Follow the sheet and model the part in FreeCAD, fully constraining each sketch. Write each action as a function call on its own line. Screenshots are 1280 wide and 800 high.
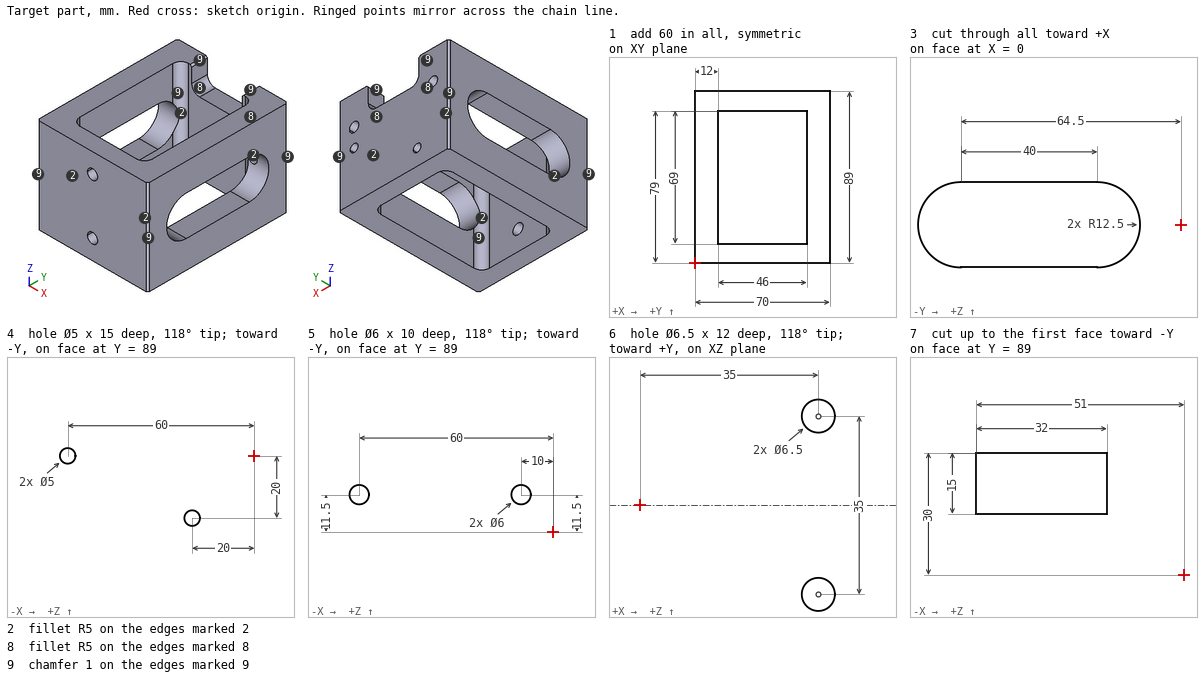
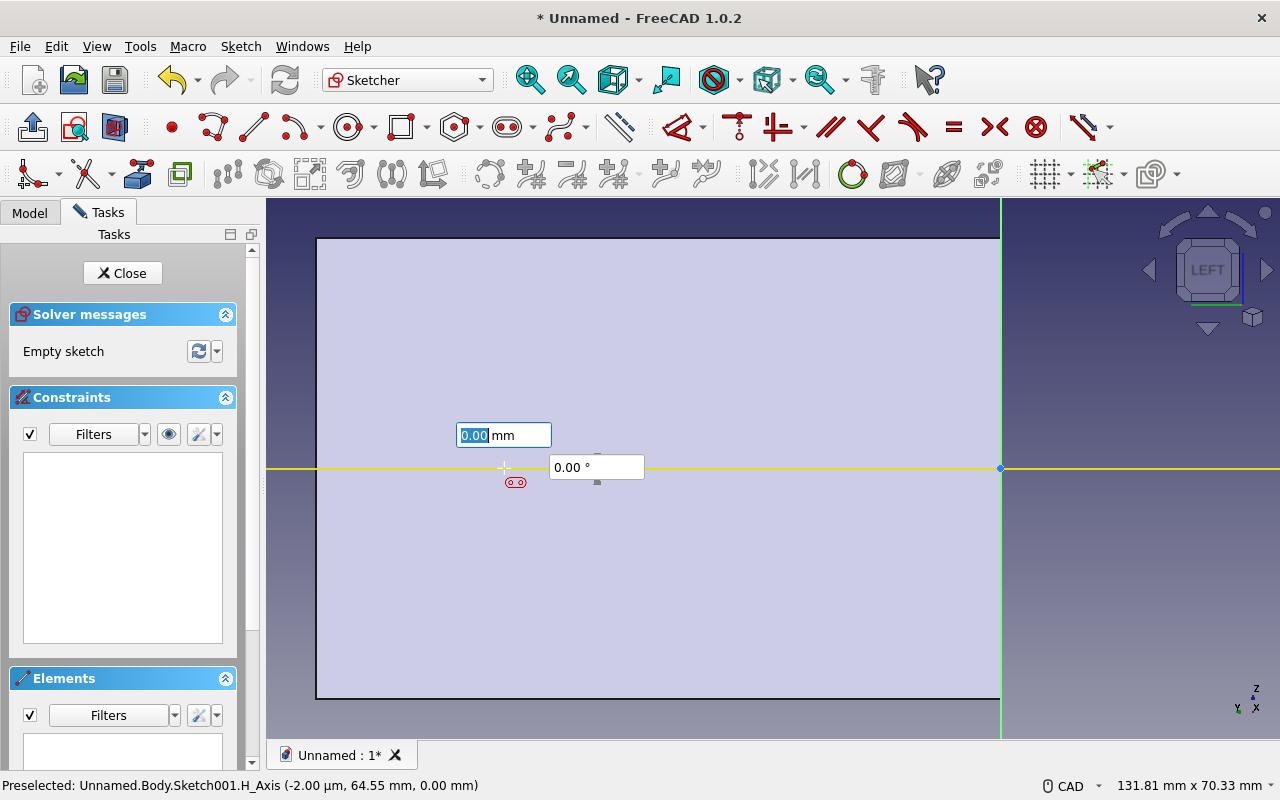
click(812, 459)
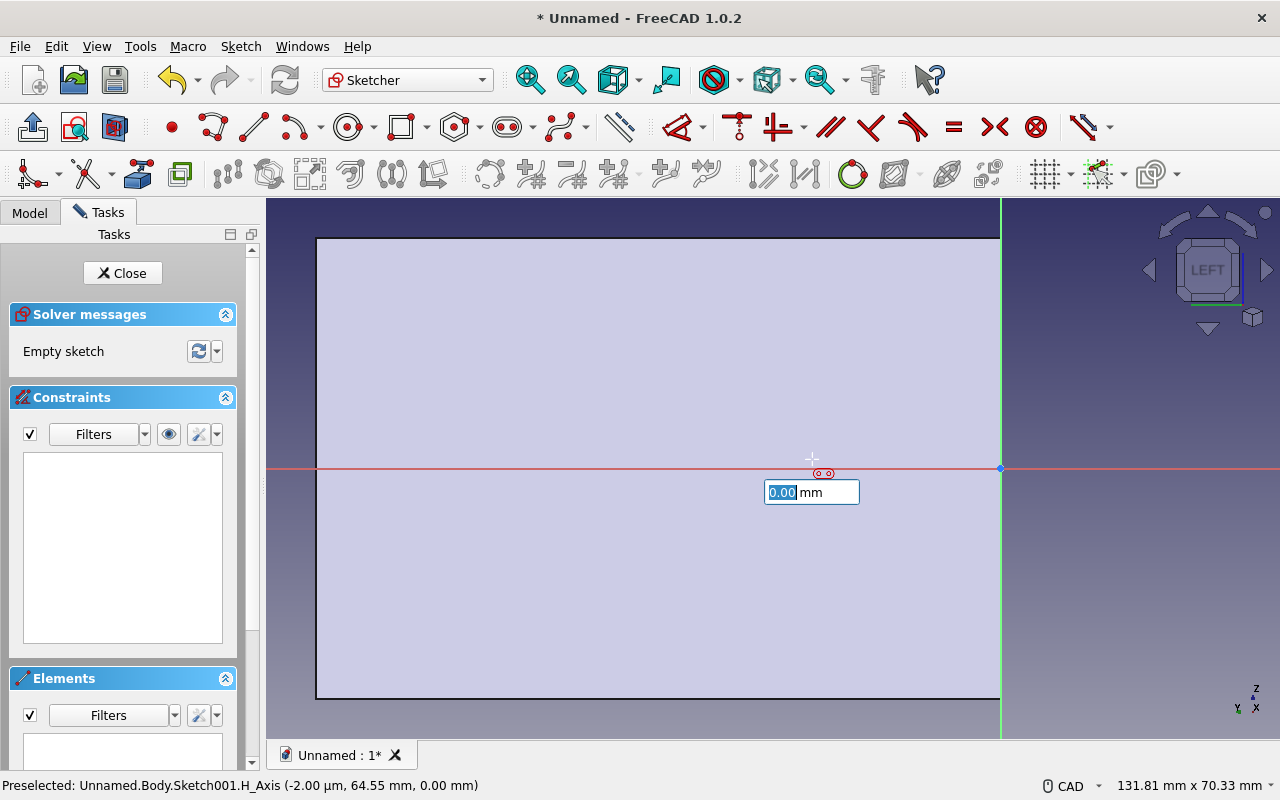
click(658, 565)
key(Escape)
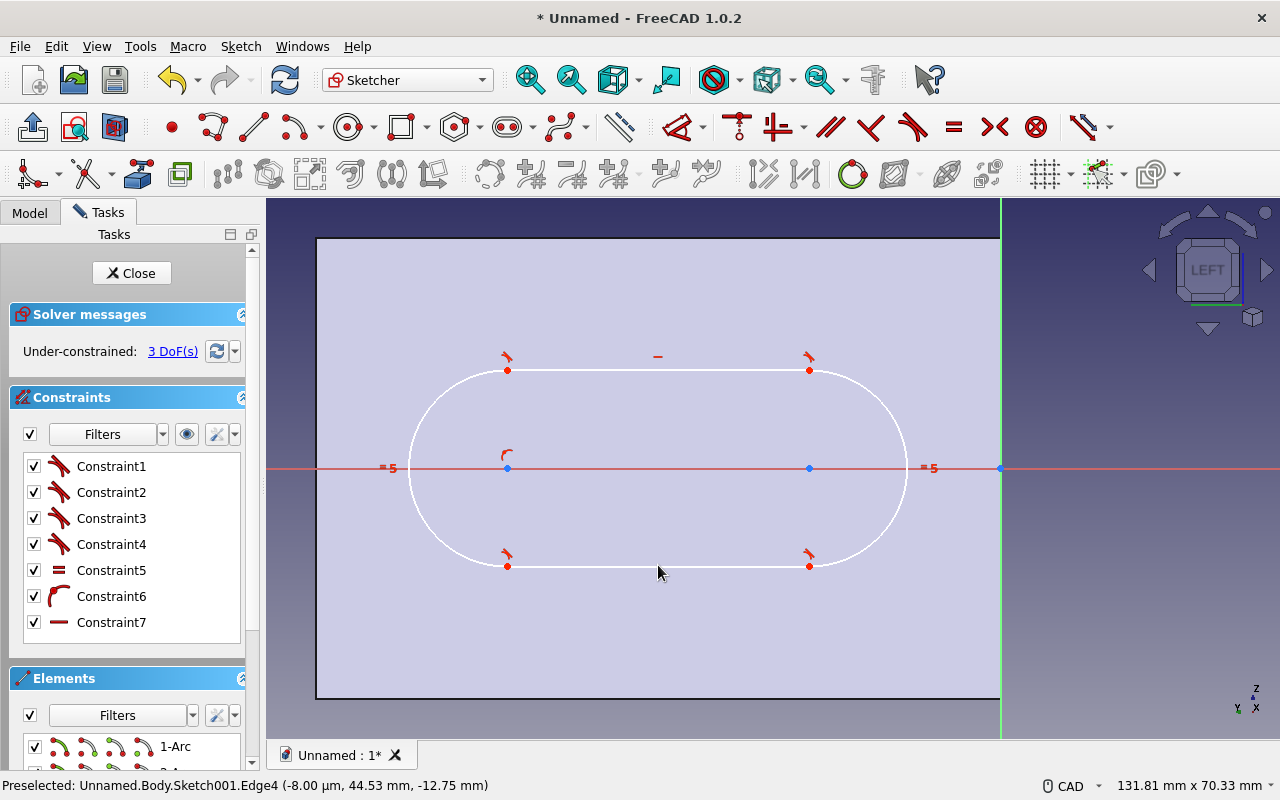
click(676, 128)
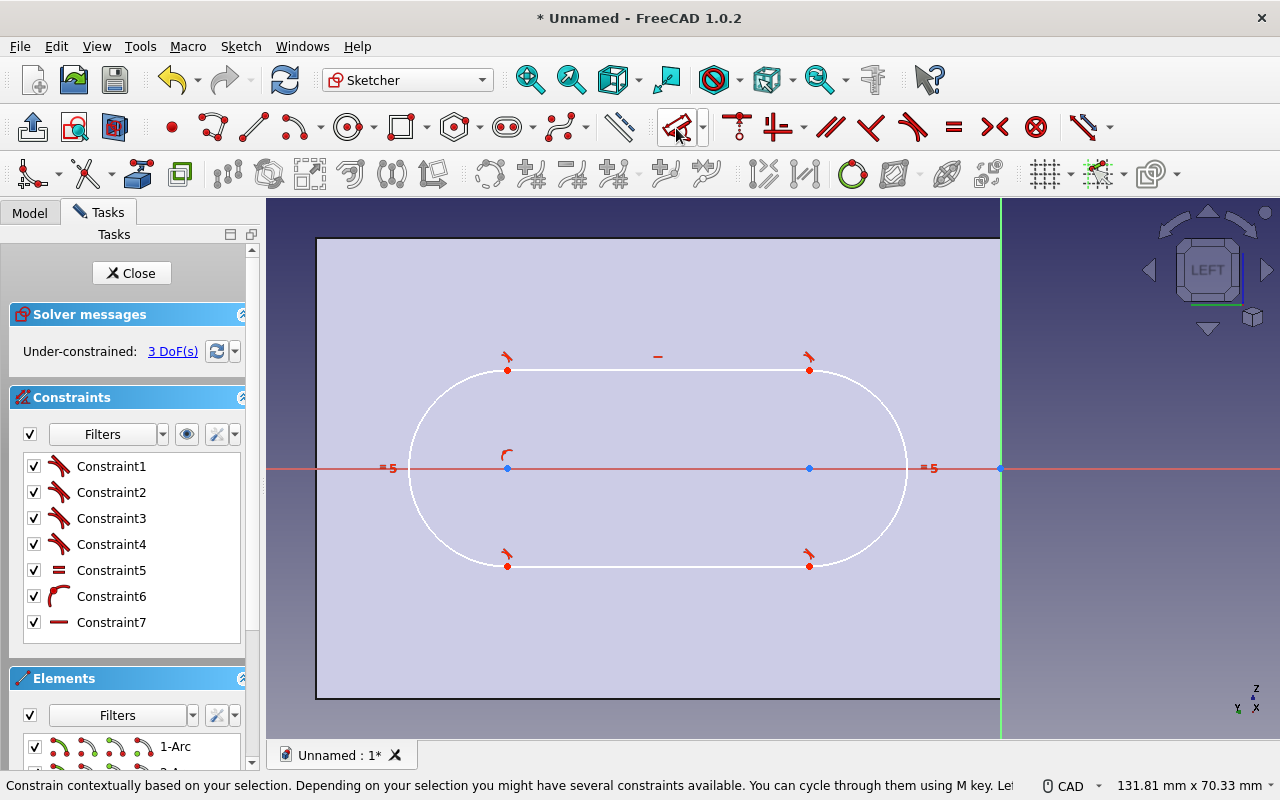
click(428, 411)
click(402, 392)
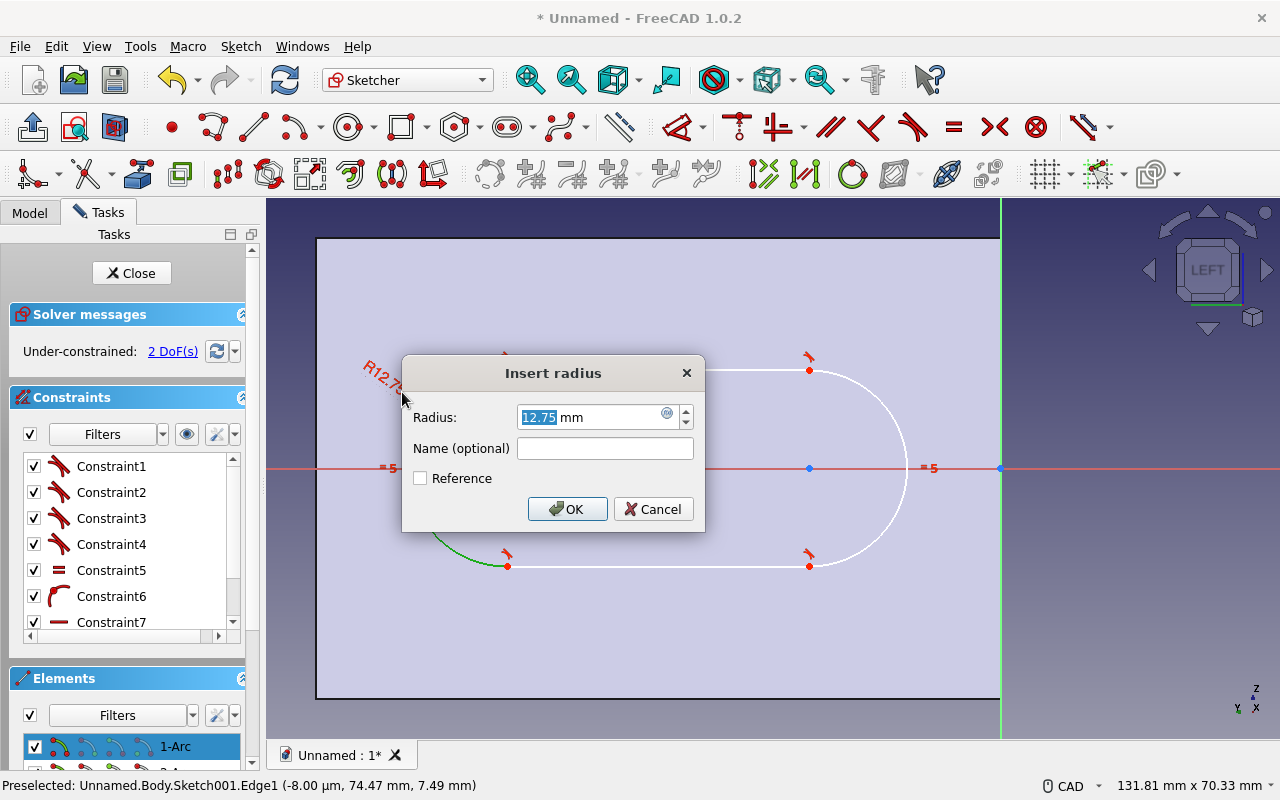
text(12.5)
key(Return)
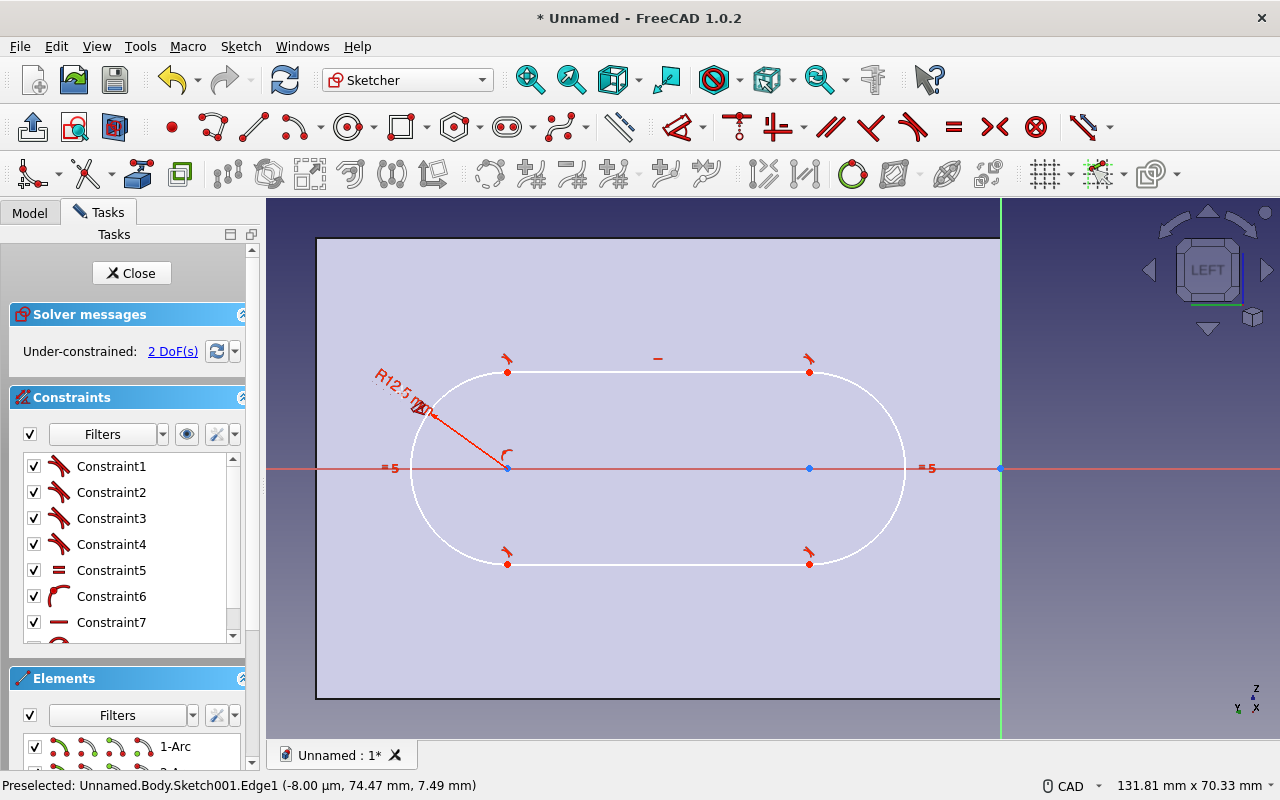
click(598, 372)
click(658, 338)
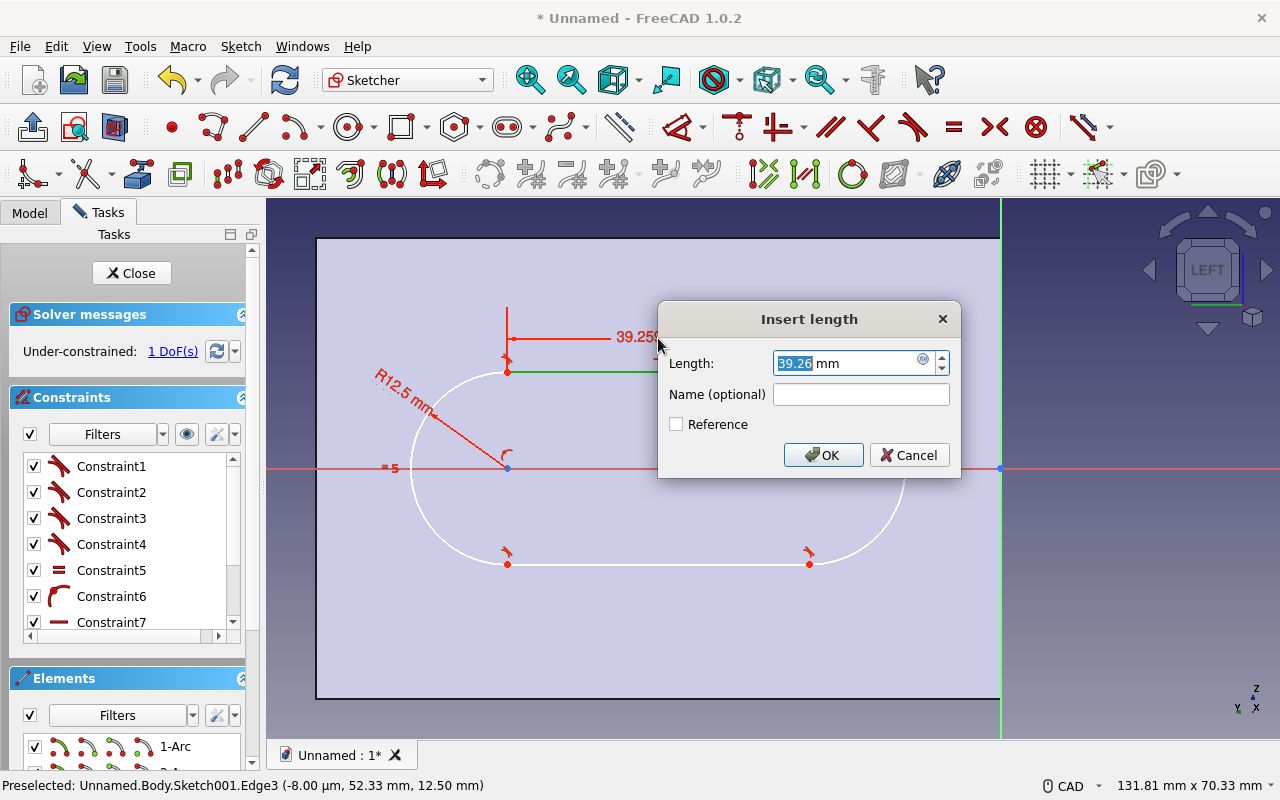
text(40)
key(Return)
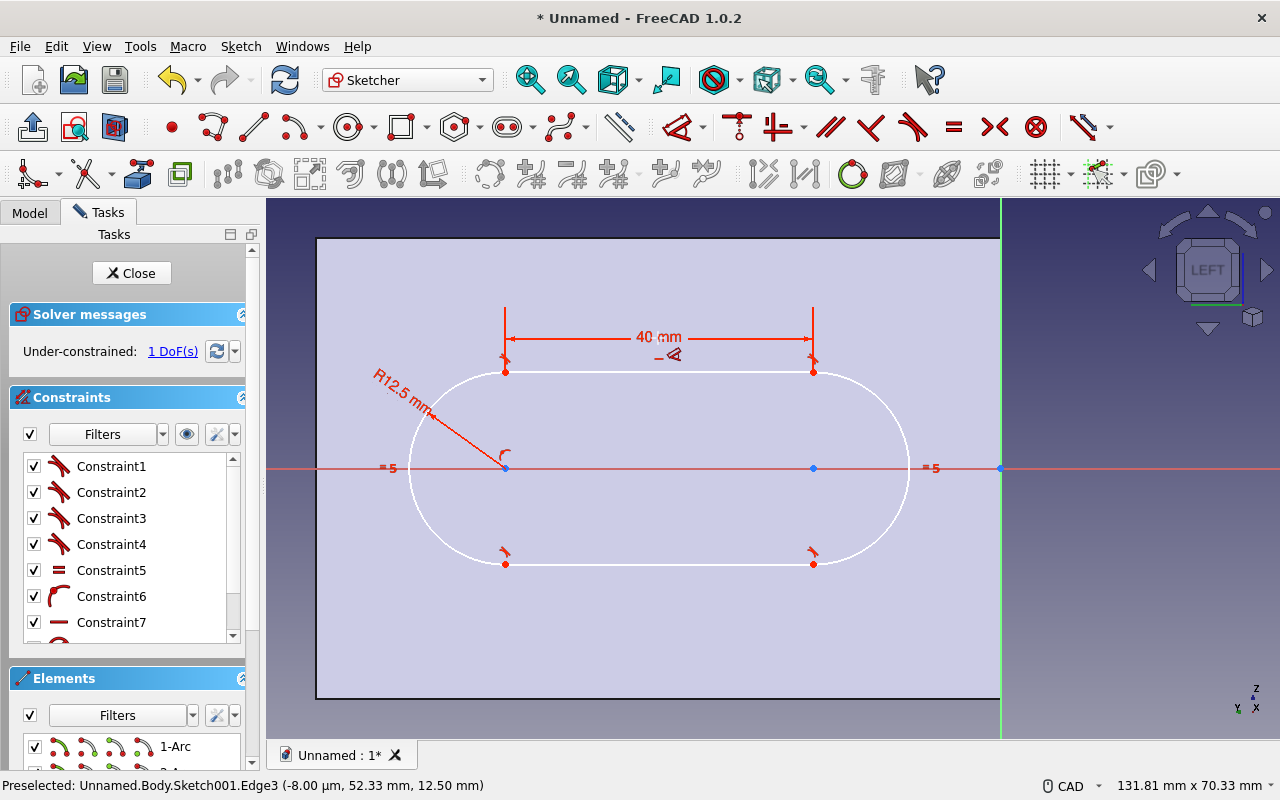
click(505, 372)
click(753, 338)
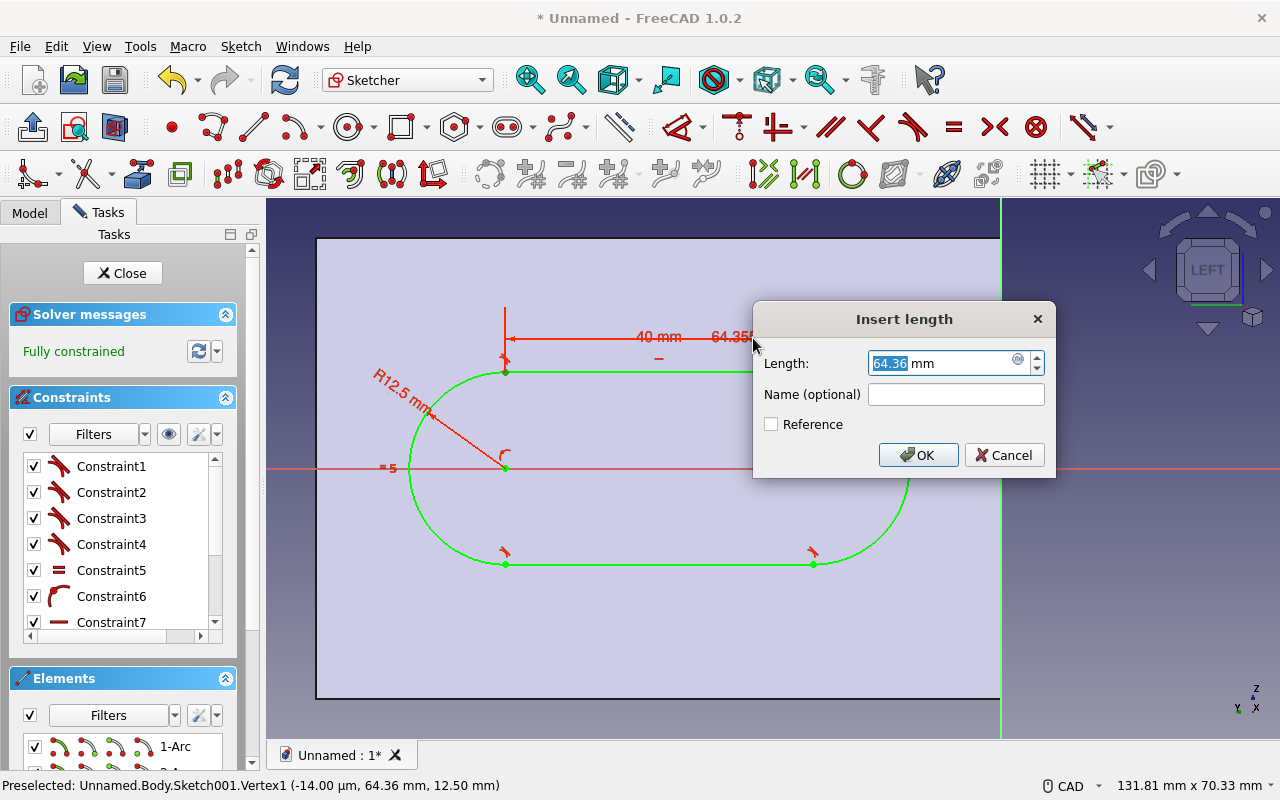
text(64.5)
key(Return)
key(Escape)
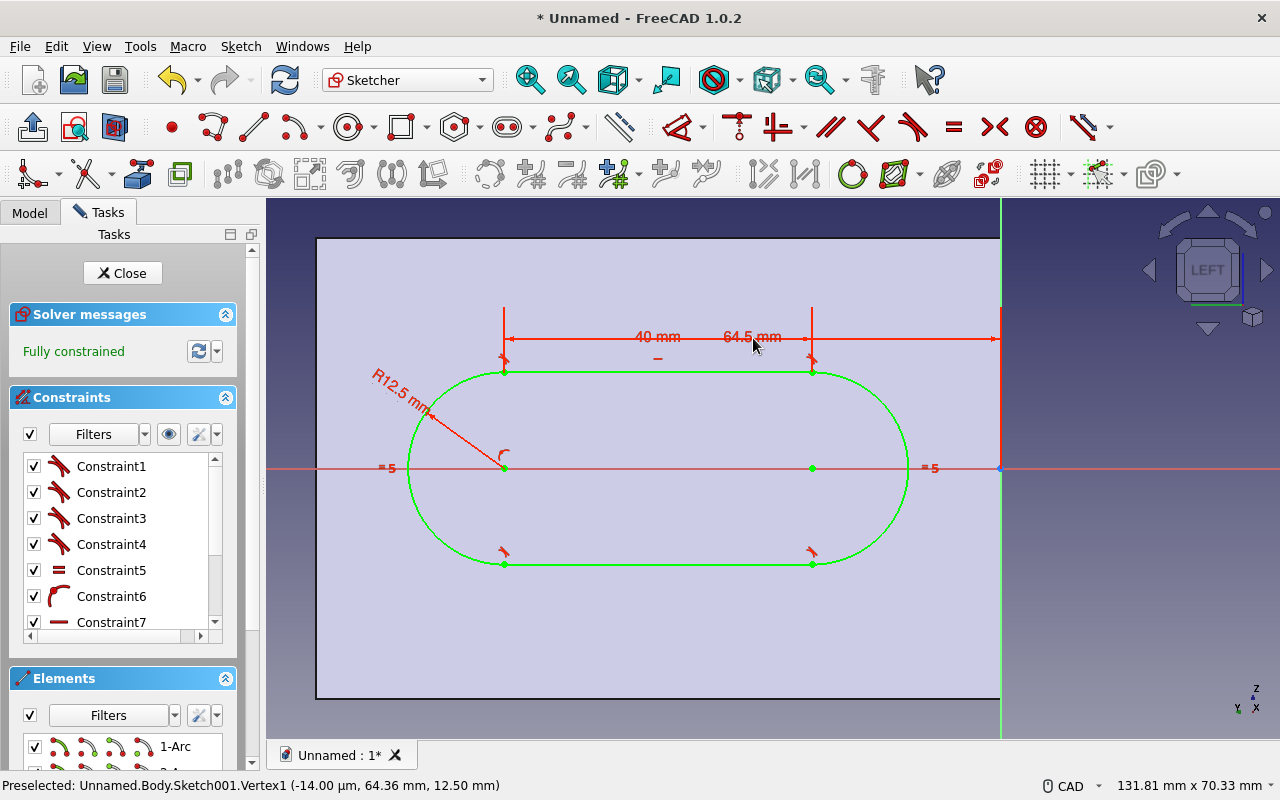
click(123, 273)